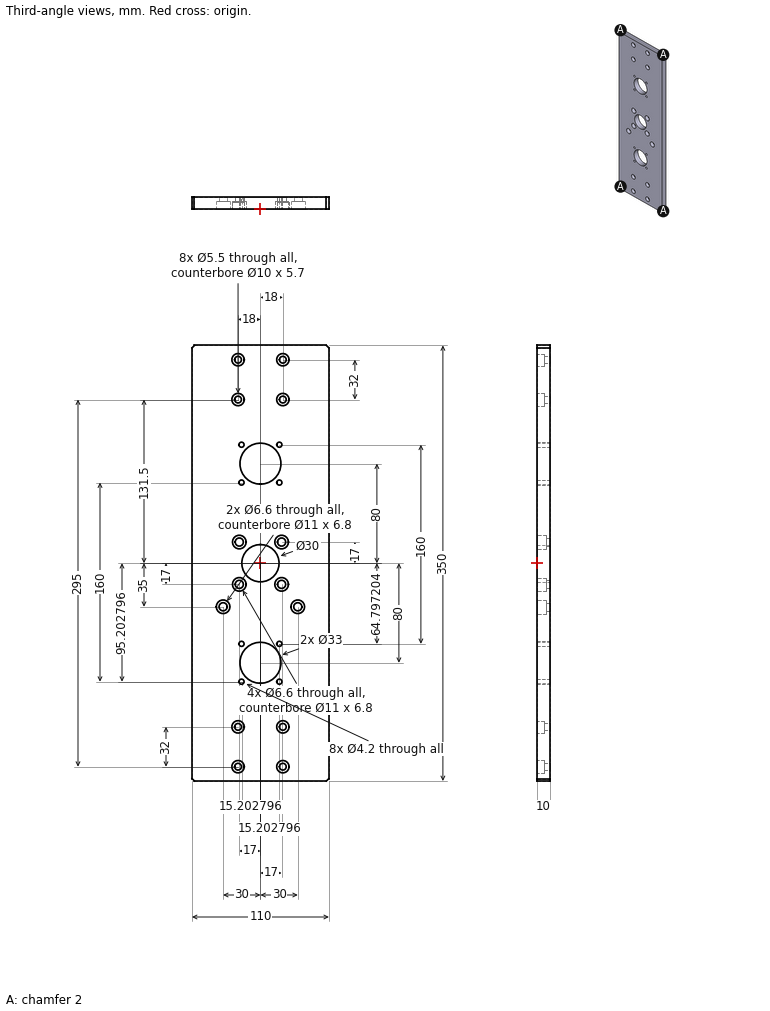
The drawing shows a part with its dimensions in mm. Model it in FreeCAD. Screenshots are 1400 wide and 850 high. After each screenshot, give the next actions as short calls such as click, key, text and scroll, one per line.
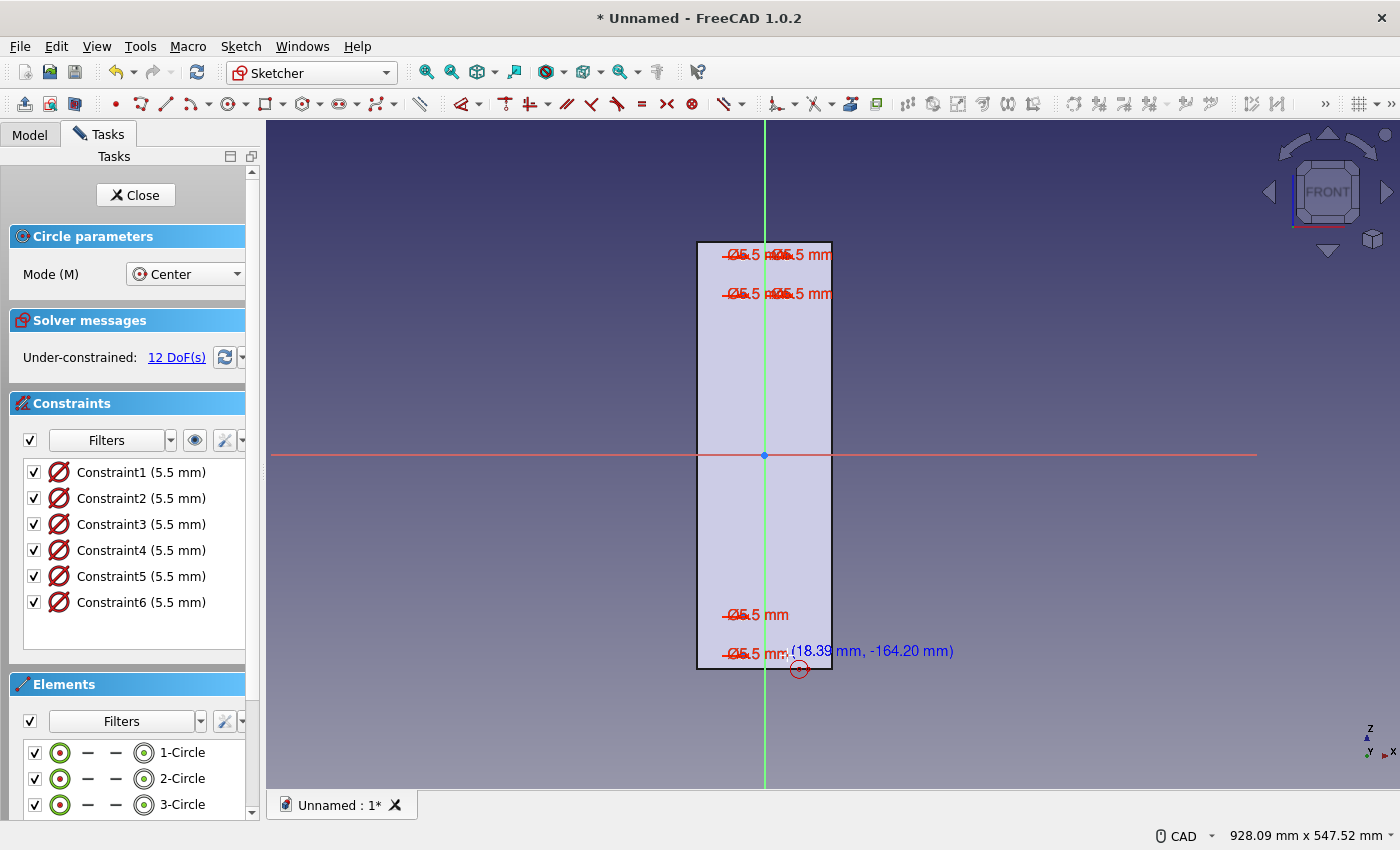
click(787, 655)
move(789, 653)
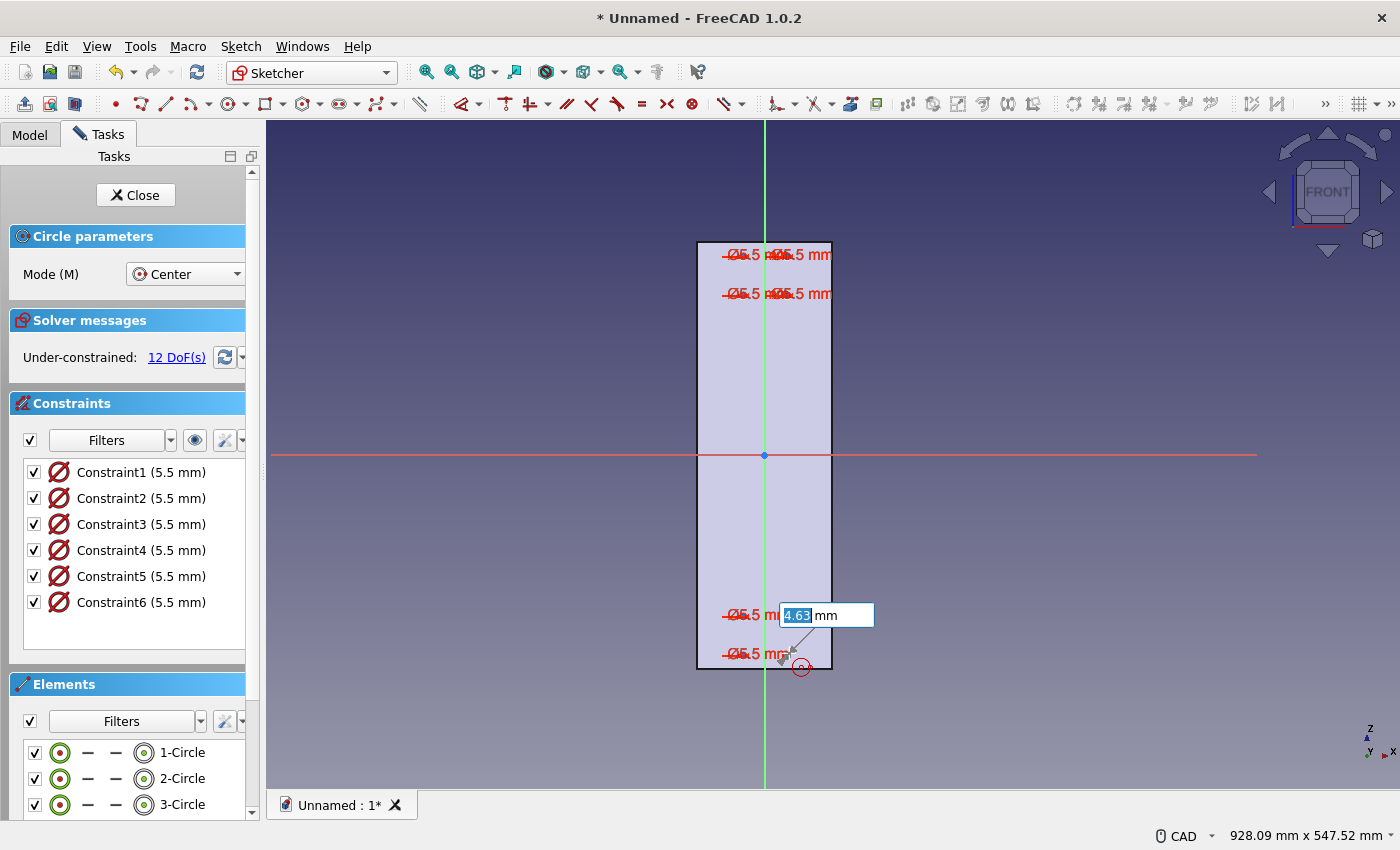
text(5.5)
key(Return)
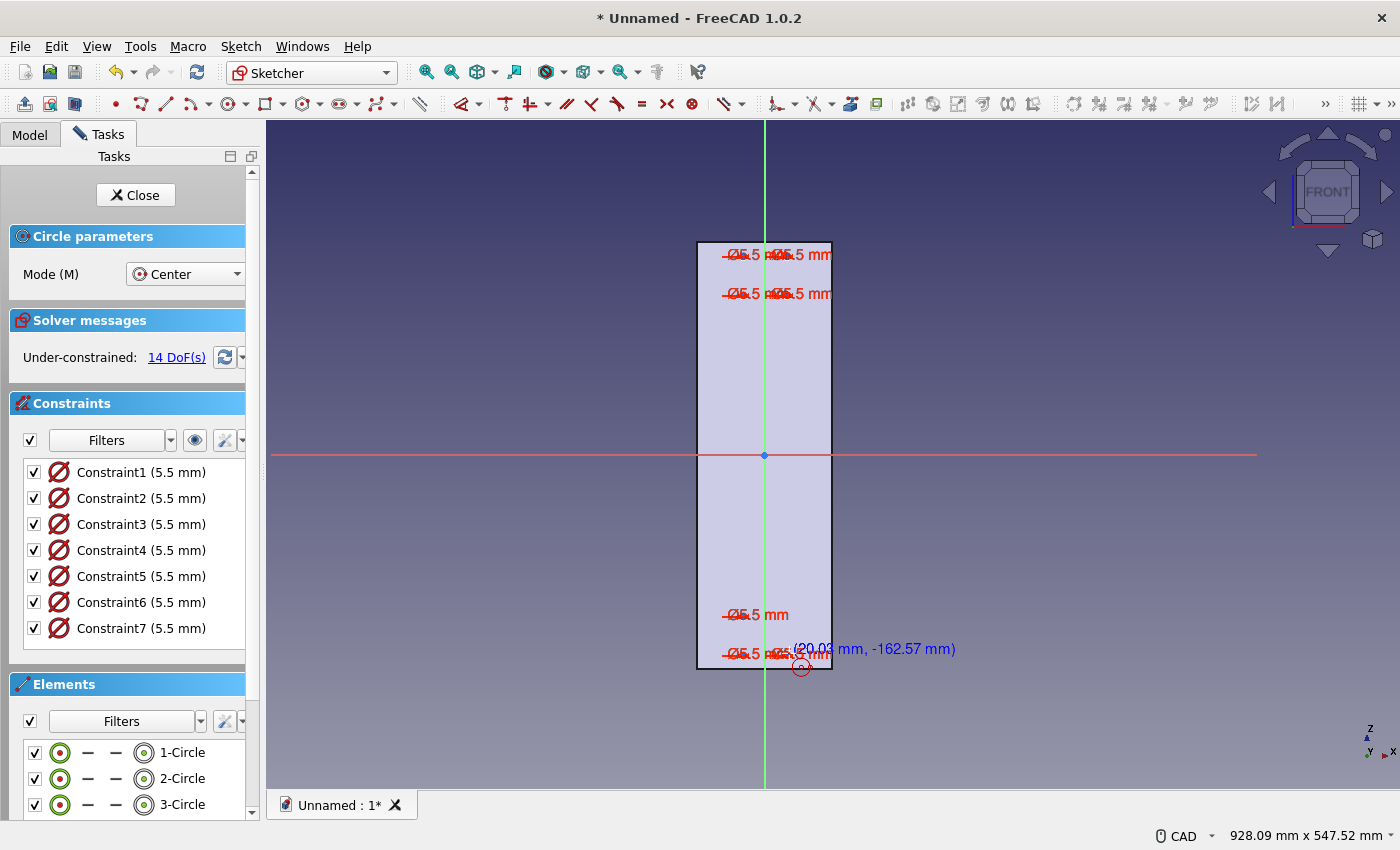
scroll(787, 616, up, 10)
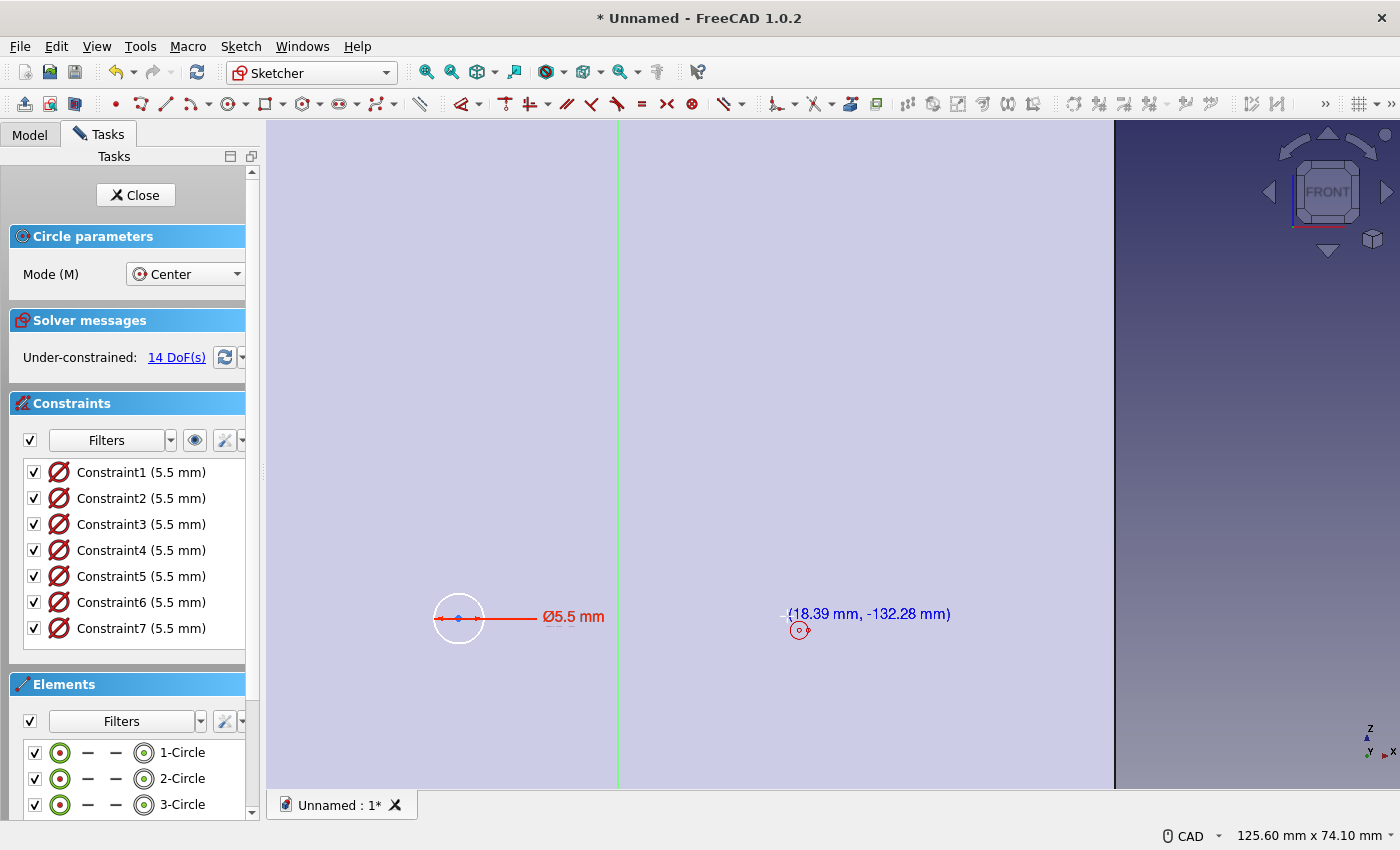
scroll(787, 616, down, 10)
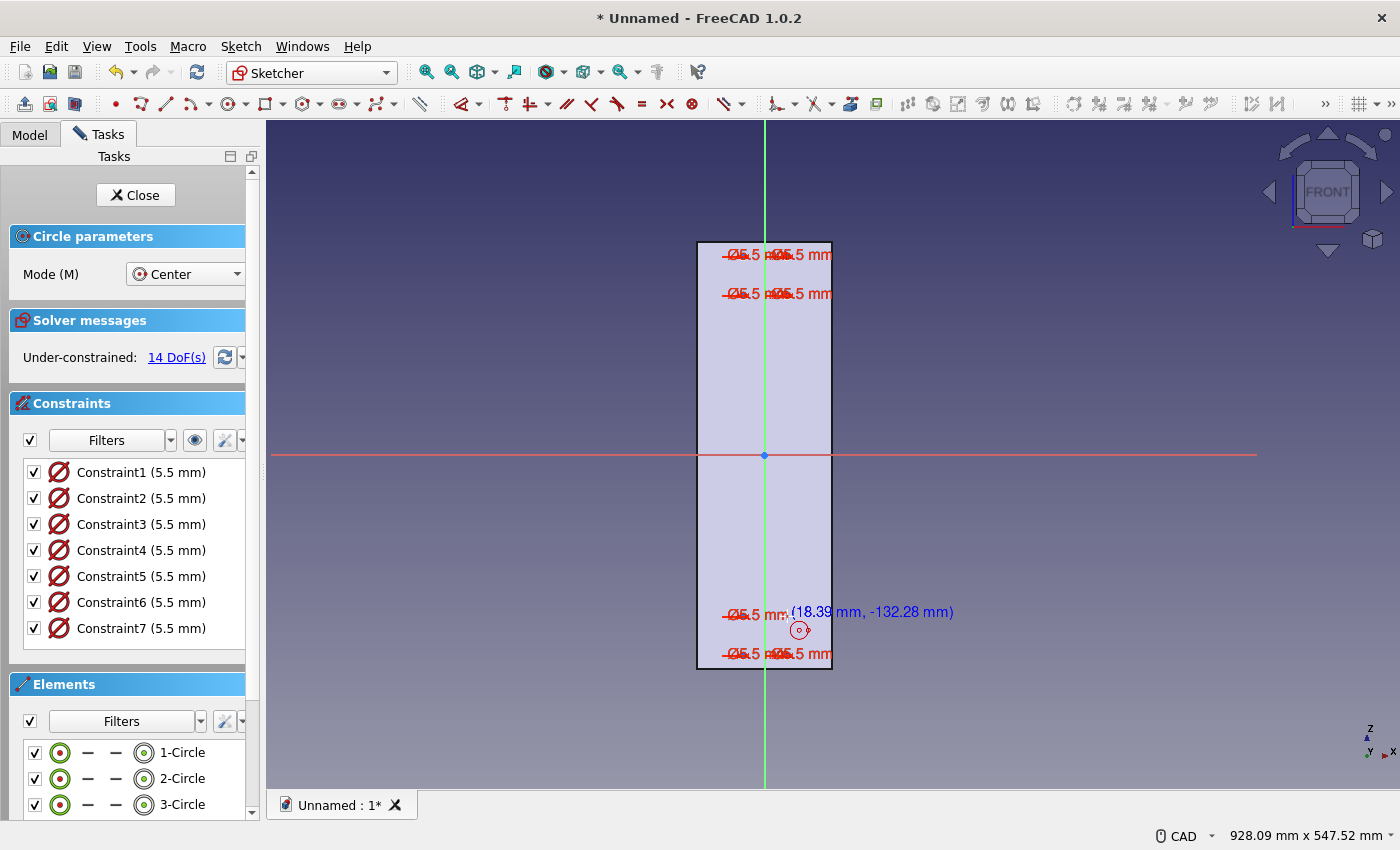
click(787, 616)
move(789, 614)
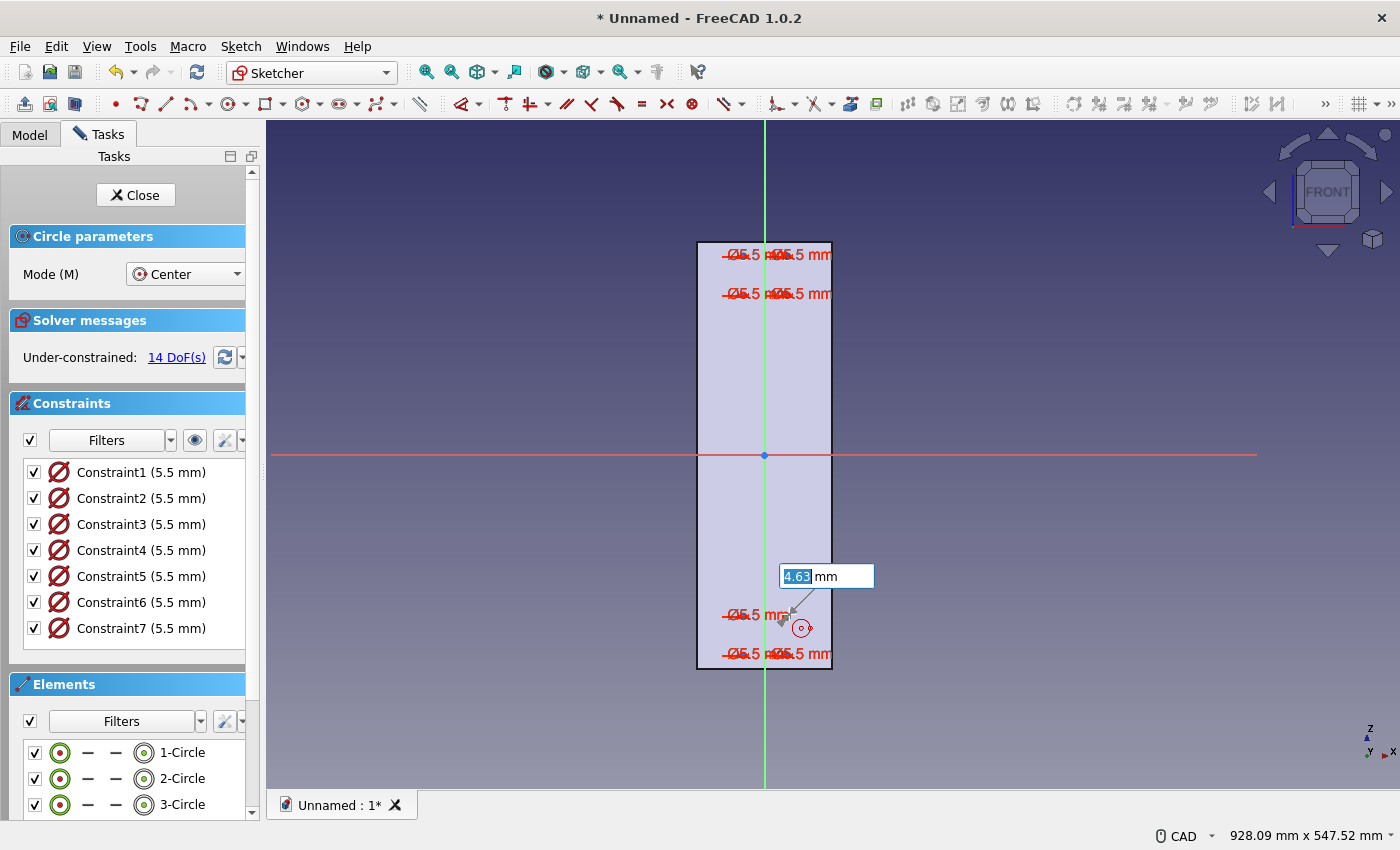
text(5.5)
key(Return)
key(Escape)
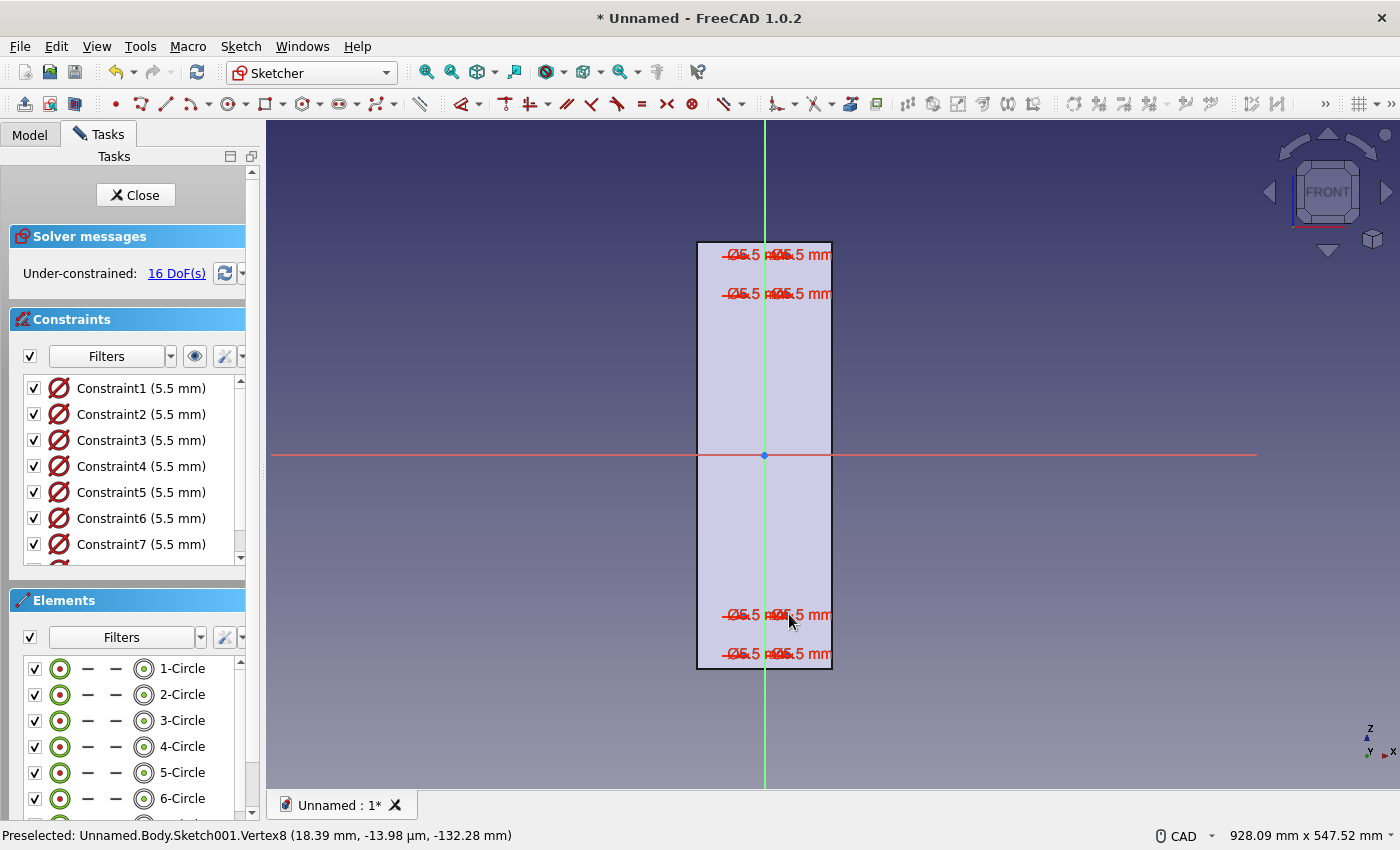
click(743, 296)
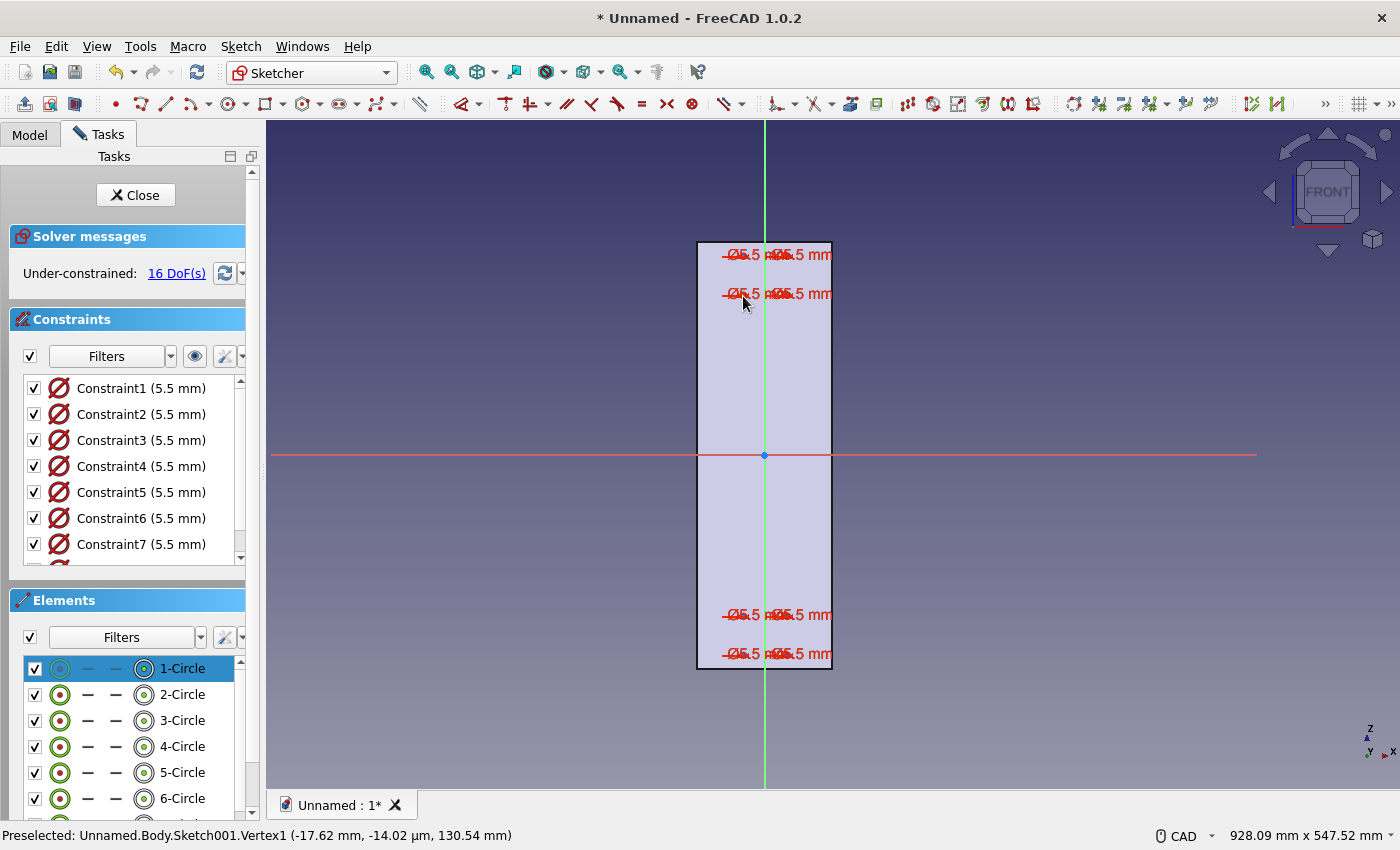
click(787, 296)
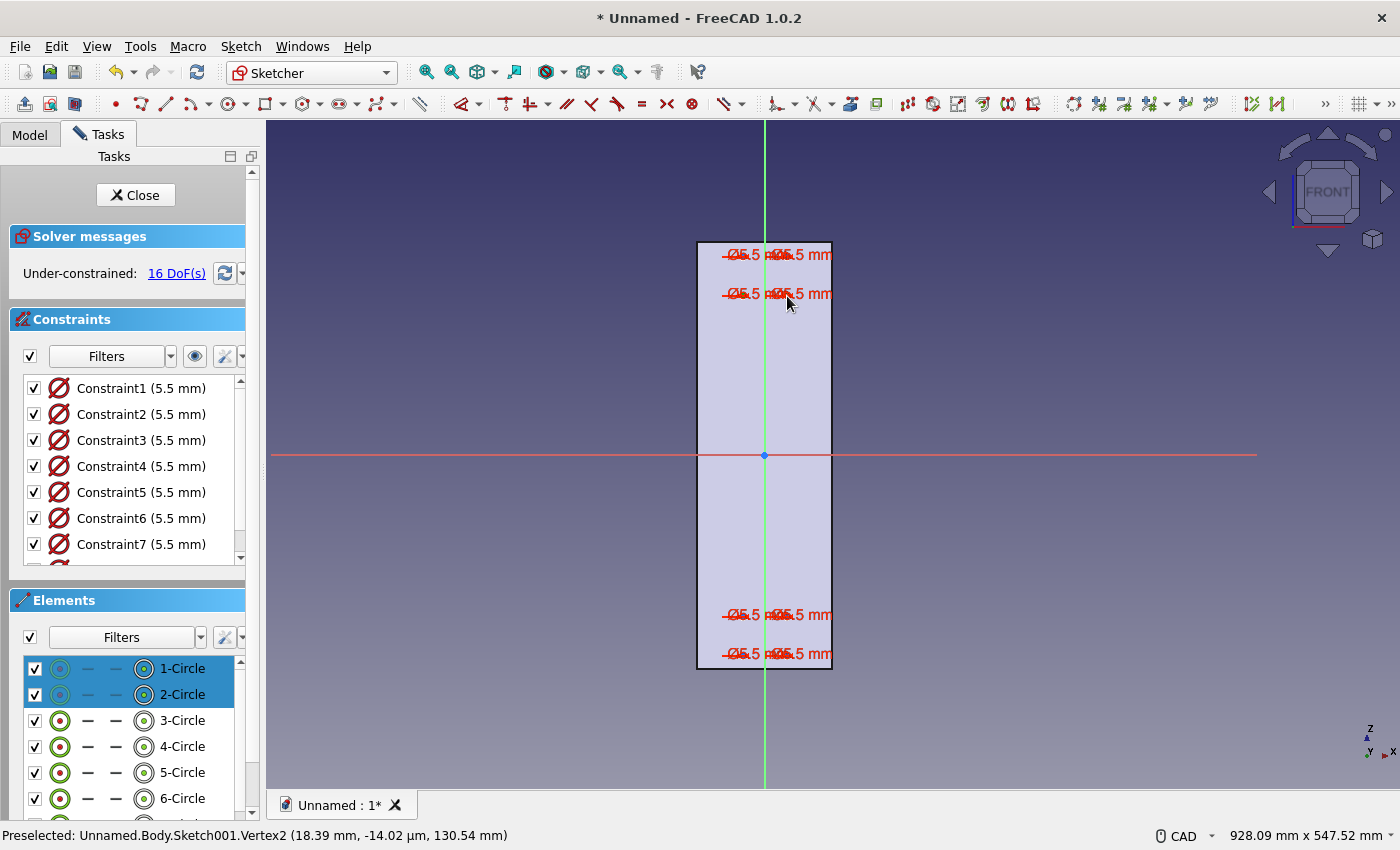
click(548, 104)